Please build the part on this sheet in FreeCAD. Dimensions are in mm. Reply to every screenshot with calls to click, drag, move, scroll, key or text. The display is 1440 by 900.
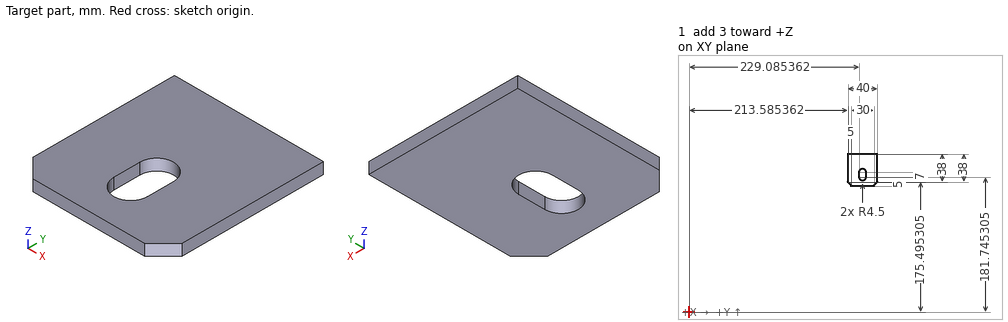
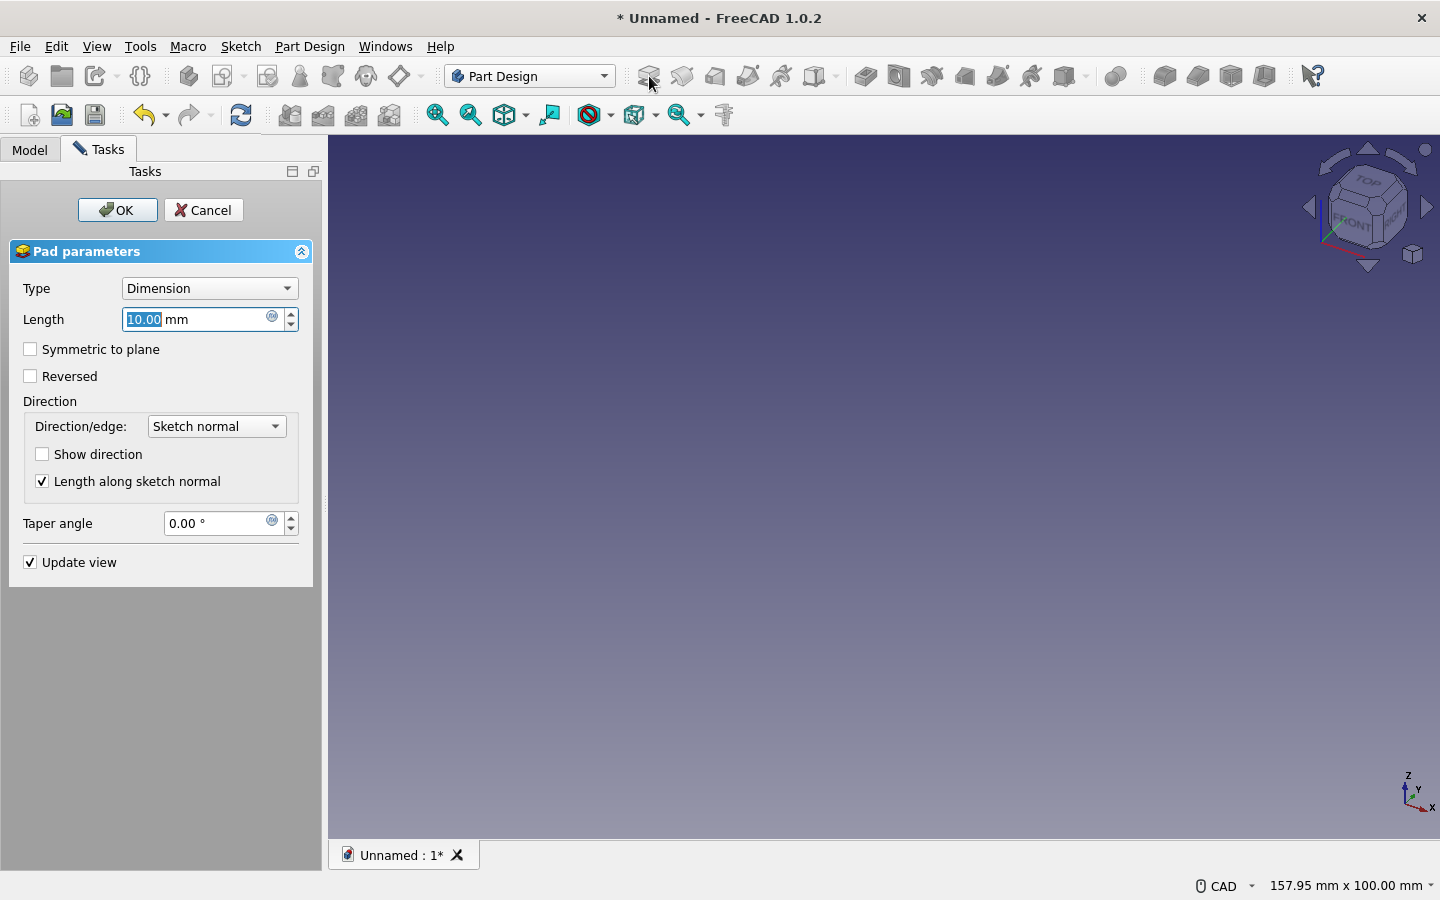
text(3)
key(Tab)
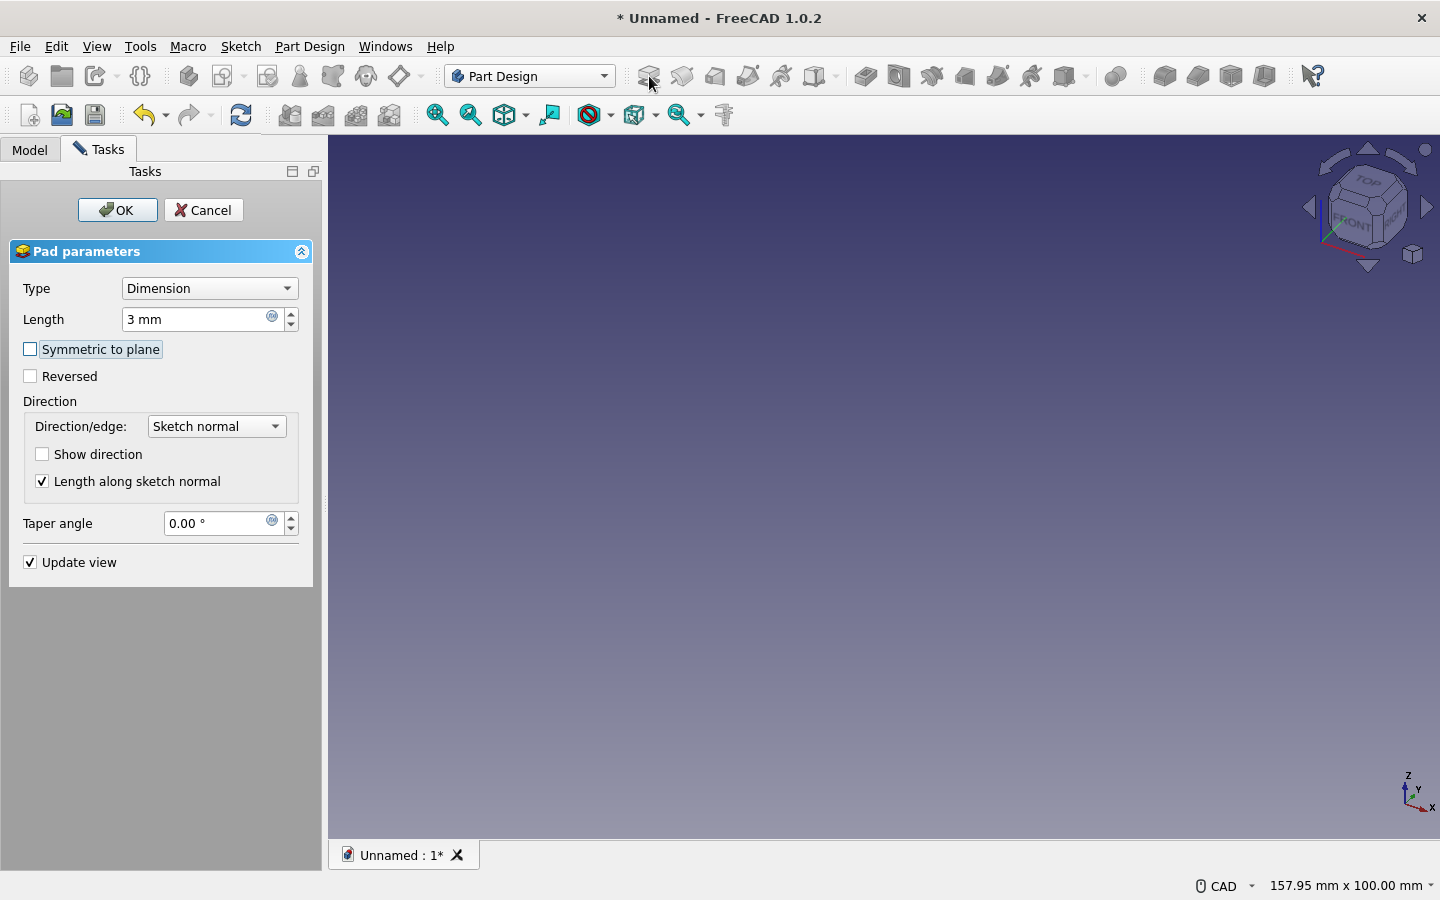
click(118, 210)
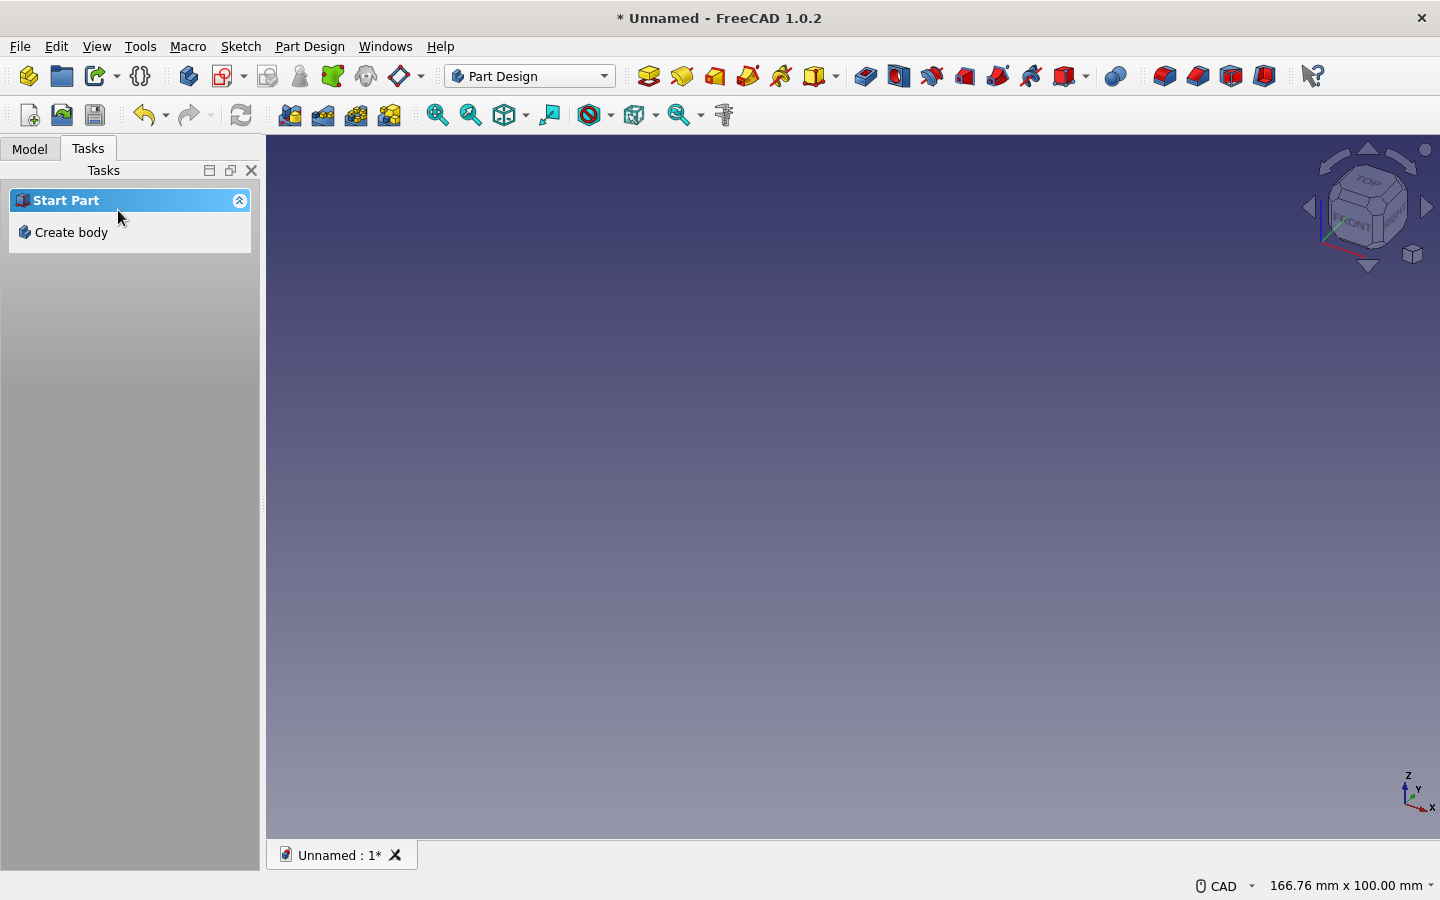
key(0)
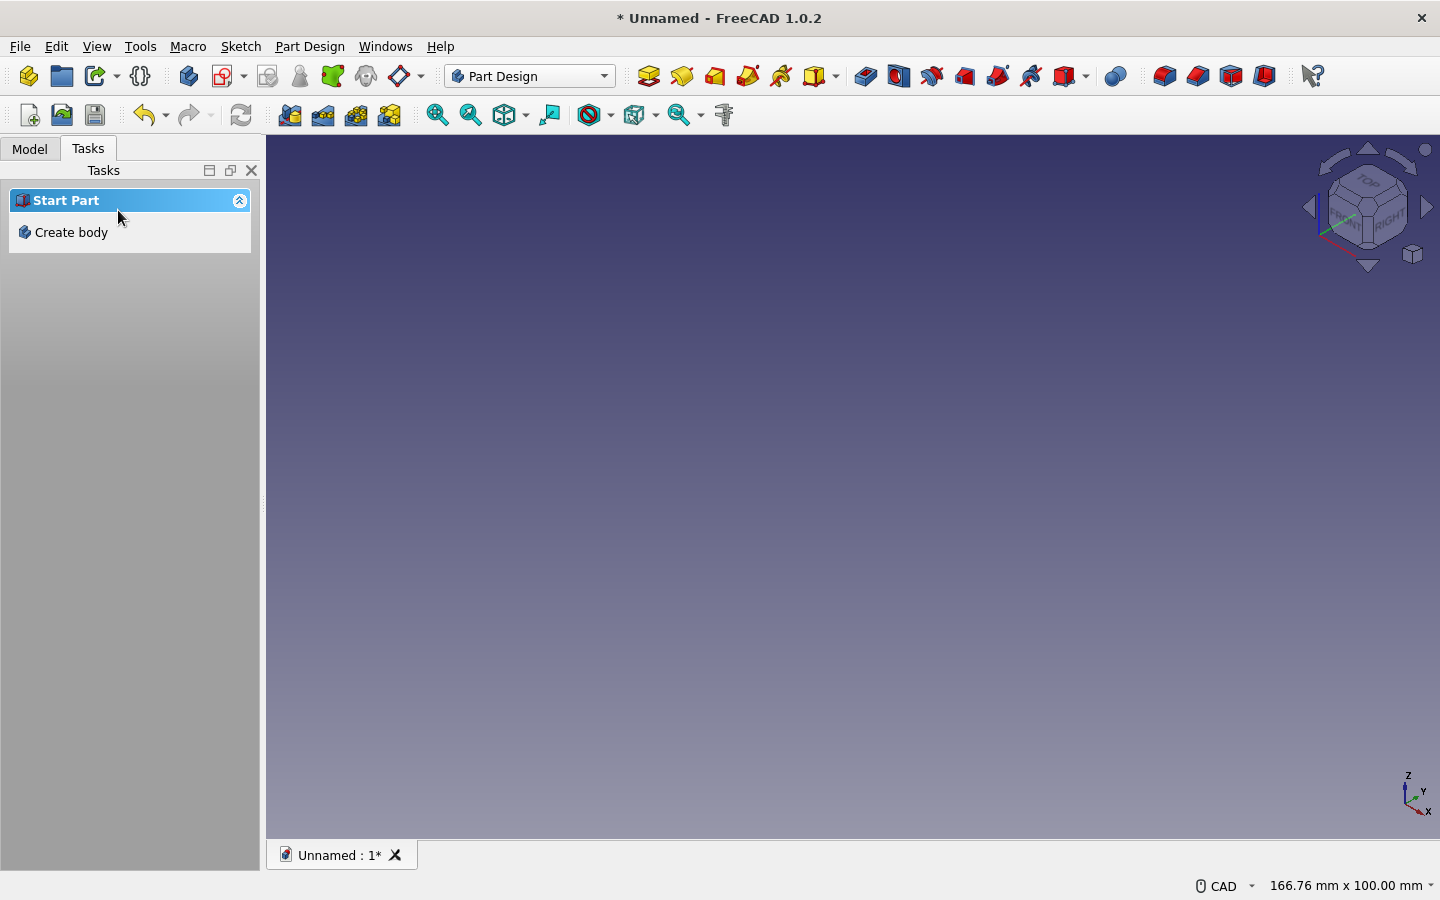
click(438, 116)